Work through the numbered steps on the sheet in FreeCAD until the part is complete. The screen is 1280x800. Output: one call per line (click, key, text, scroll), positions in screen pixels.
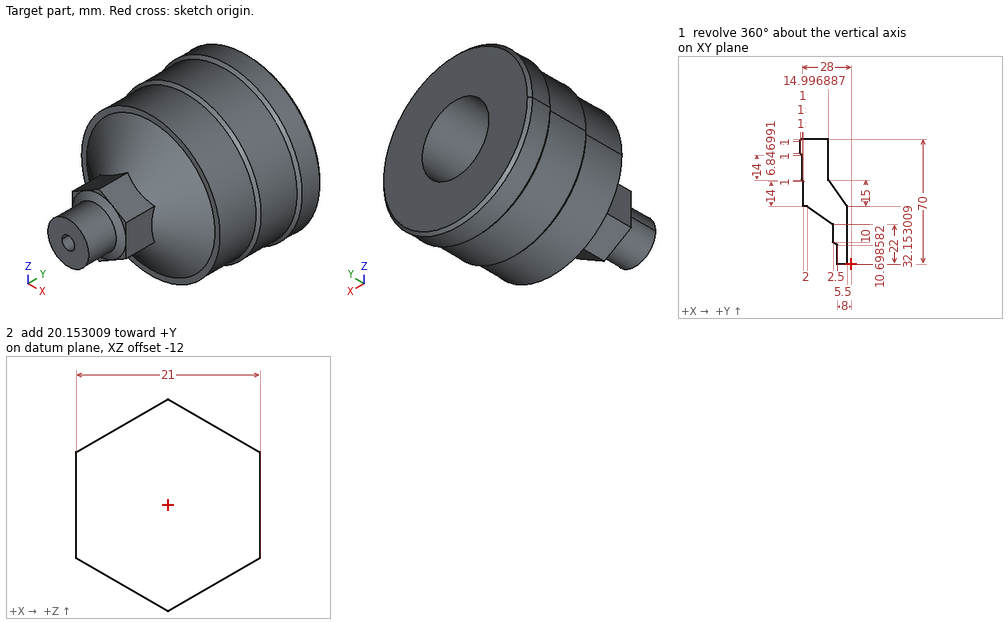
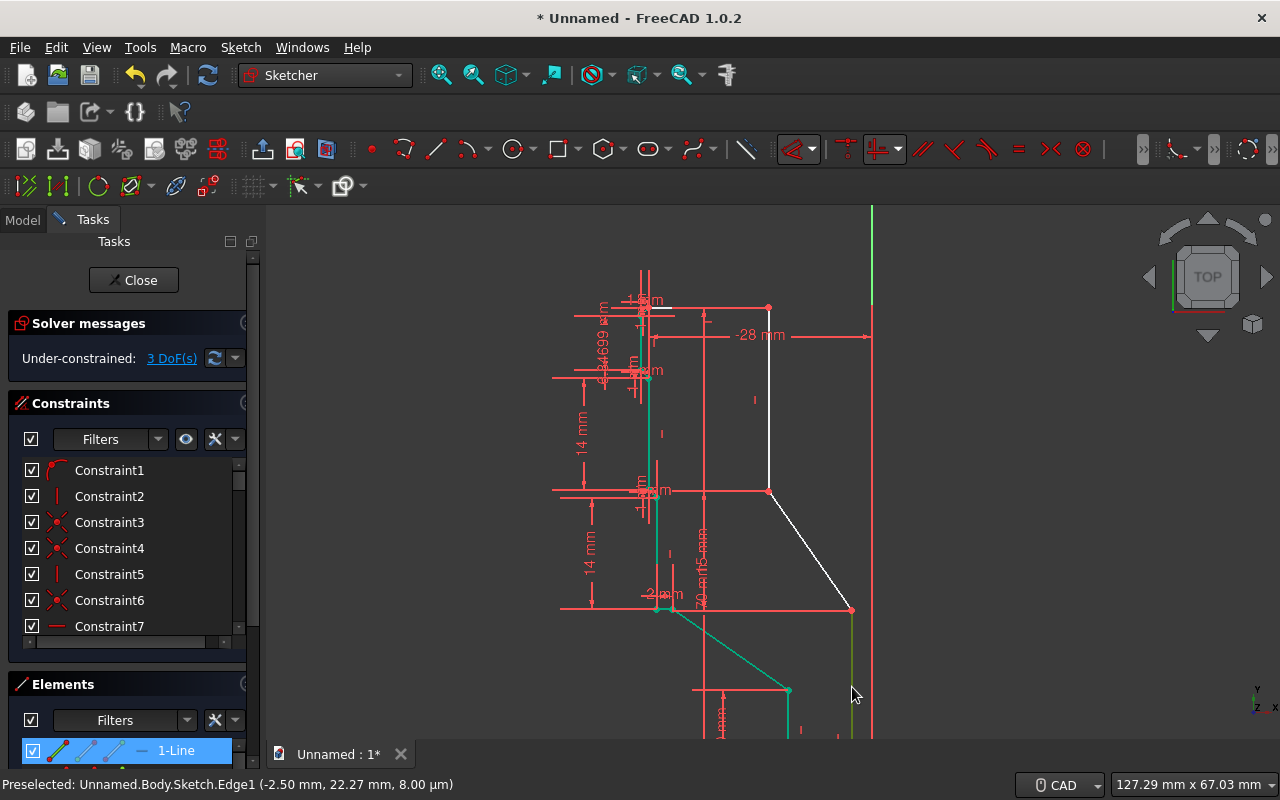
click(814, 150)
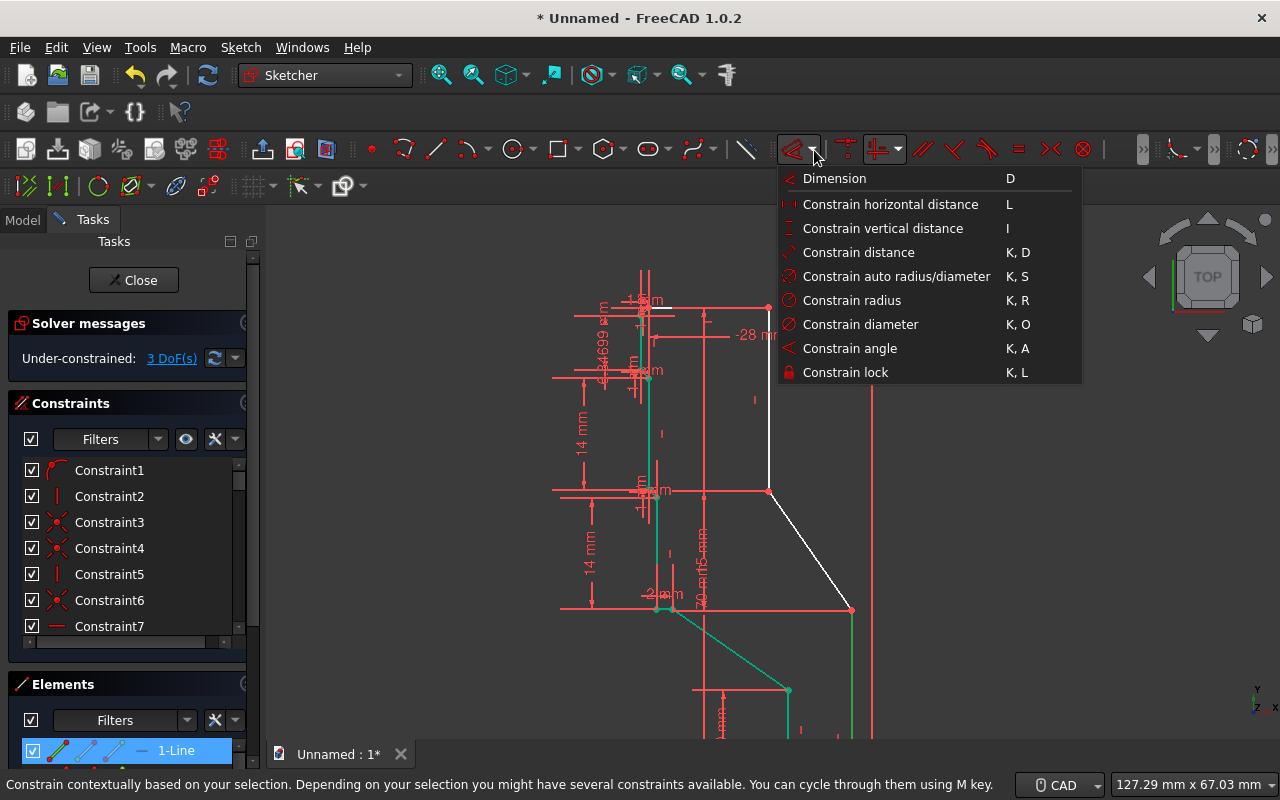
click(930, 228)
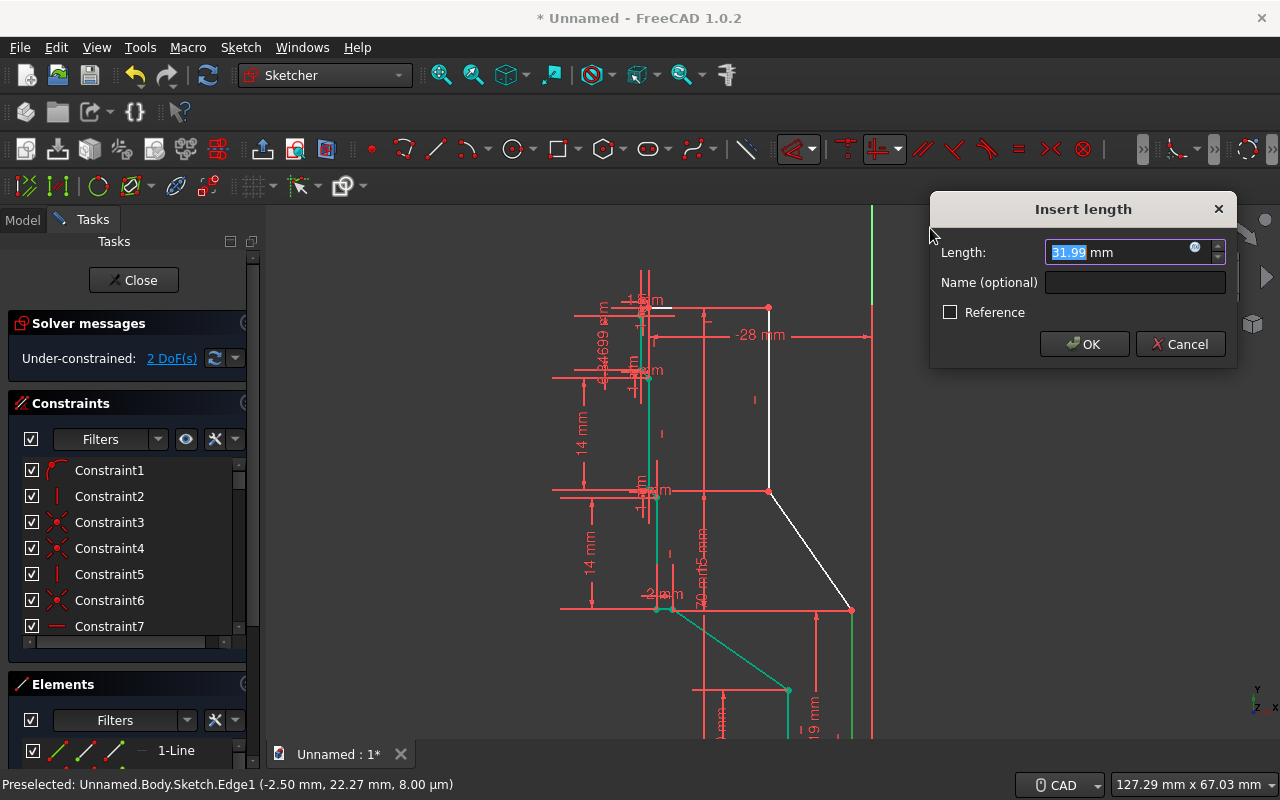
text(32.153009)
key(Return)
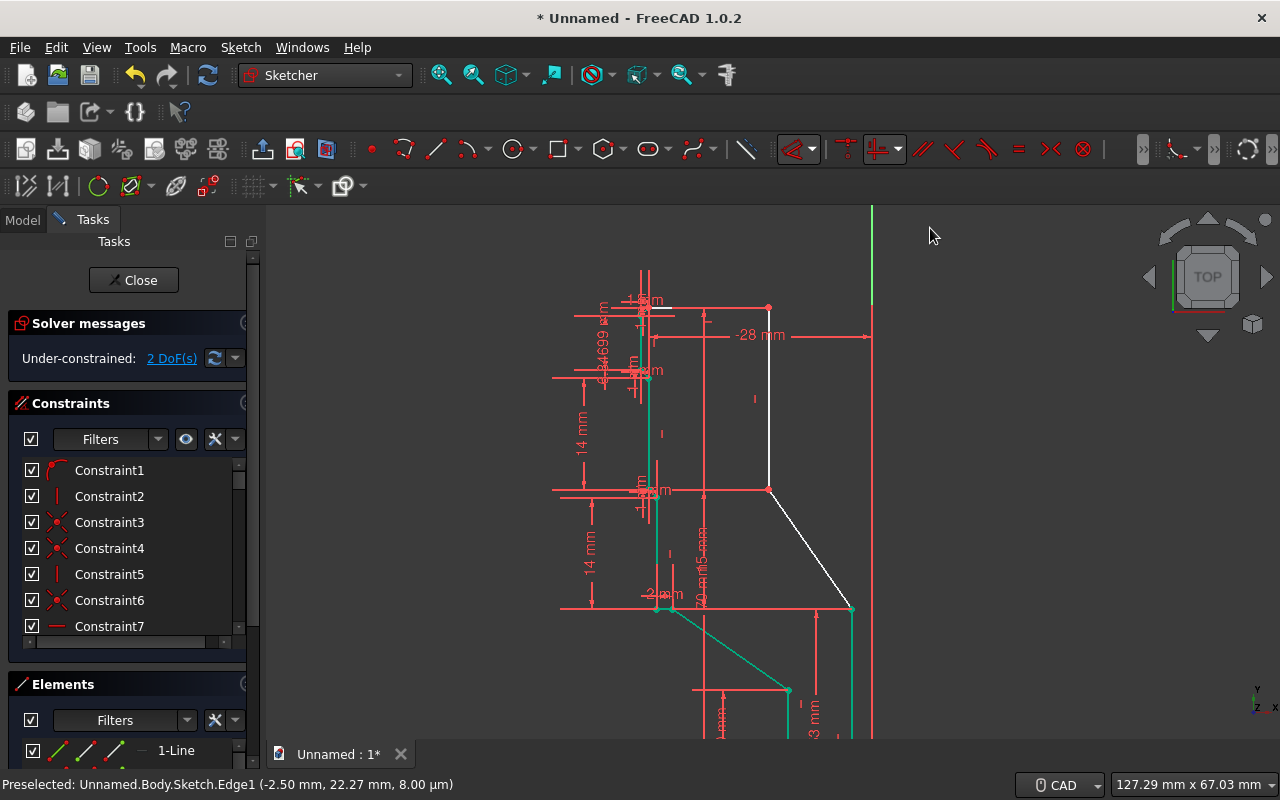
click(733, 308)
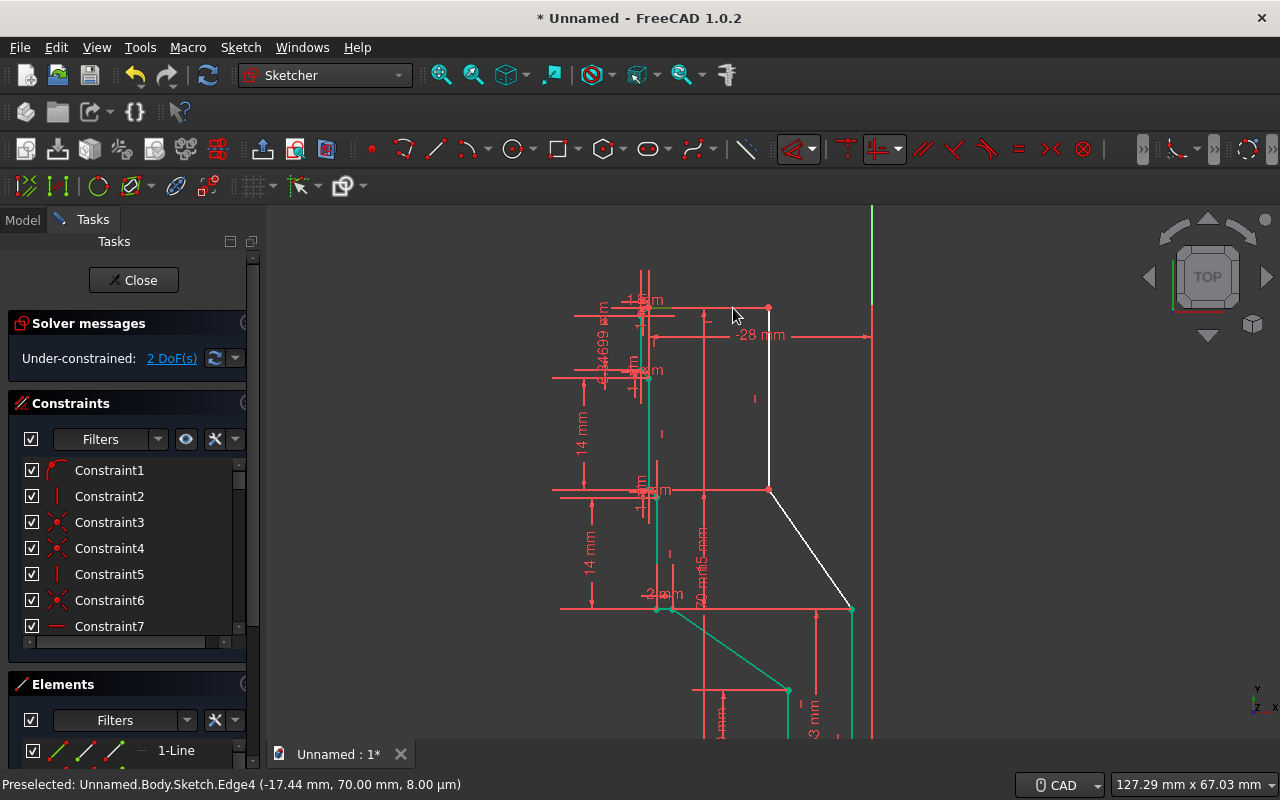
key(l)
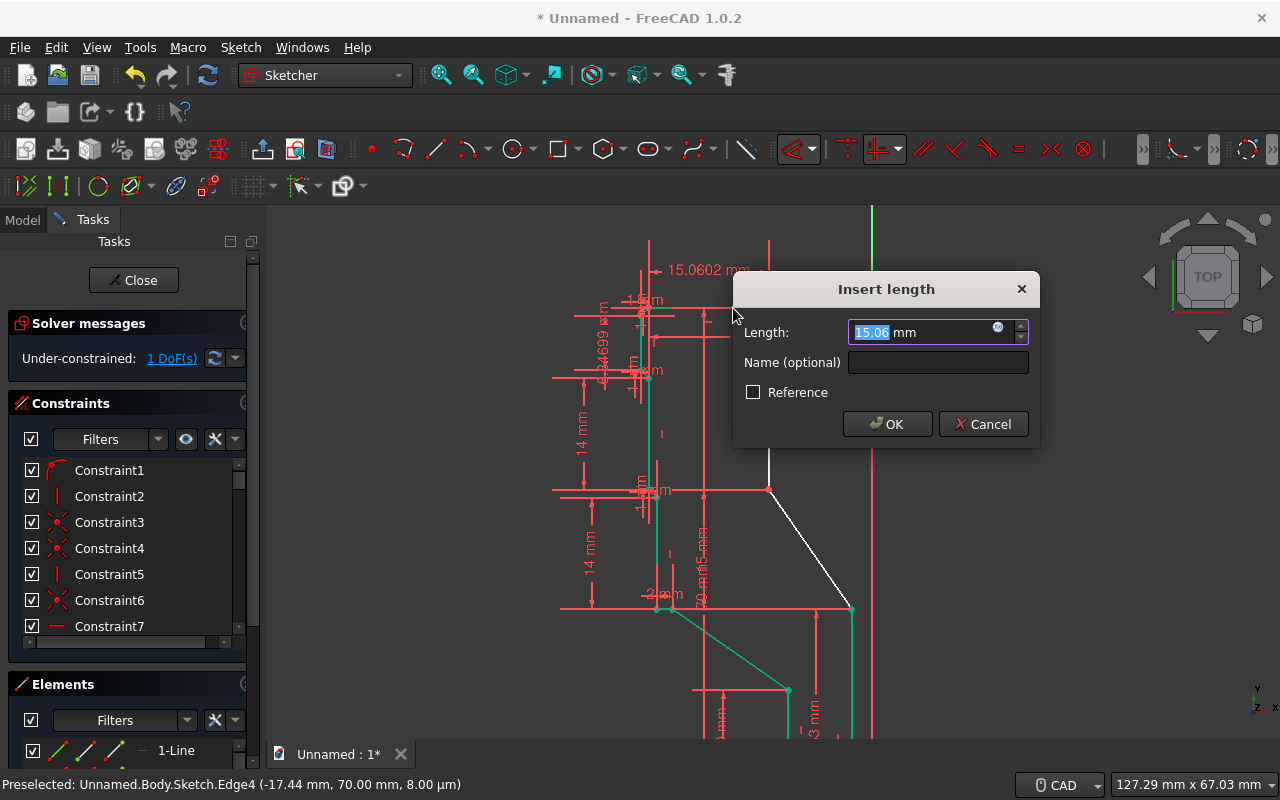
text(14.996887)
key(Return)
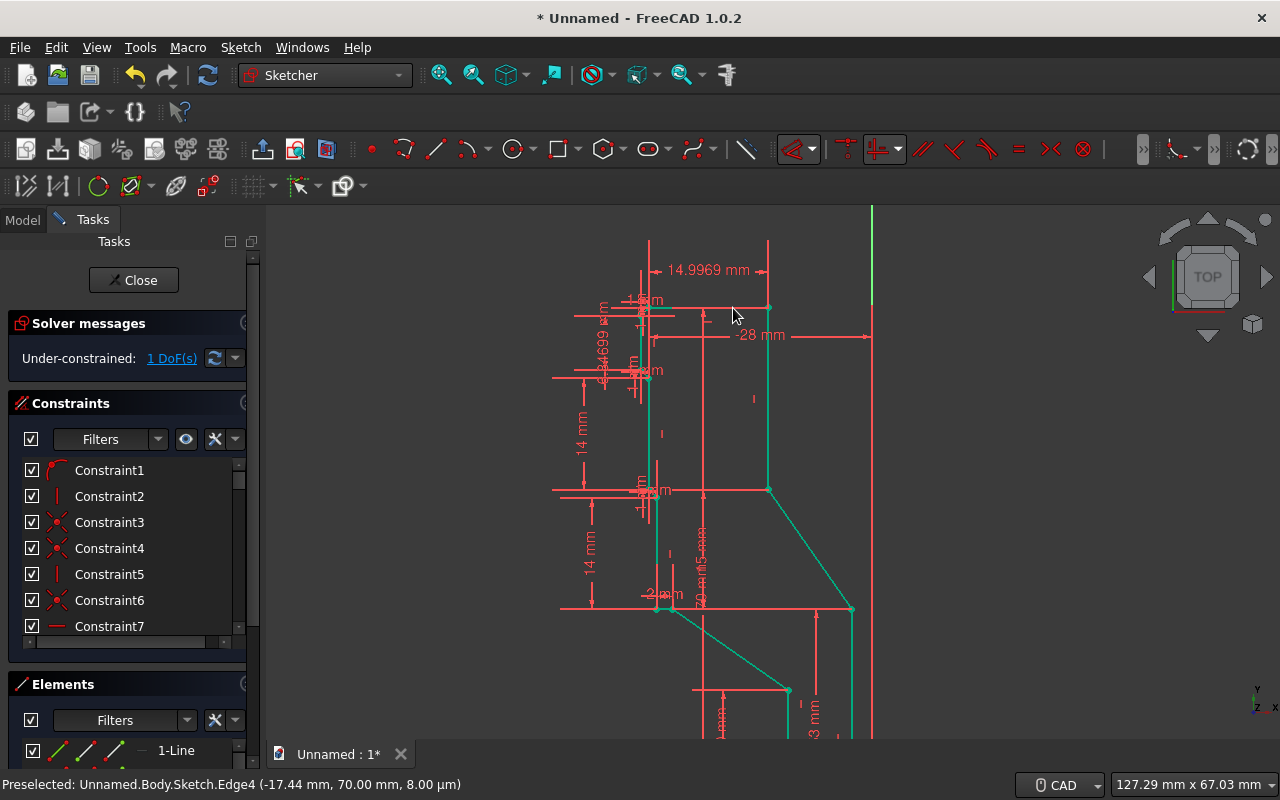
scroll(641, 333, down, 3)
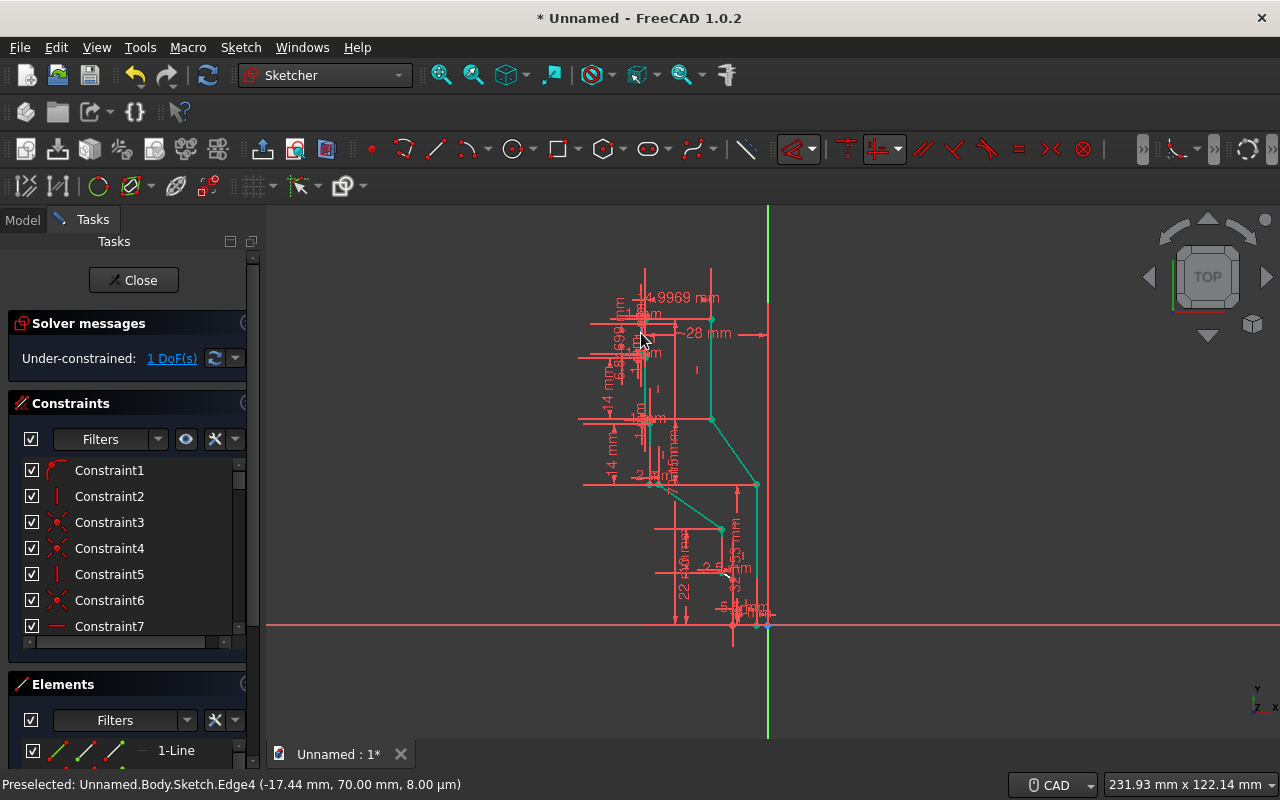
click(733, 593)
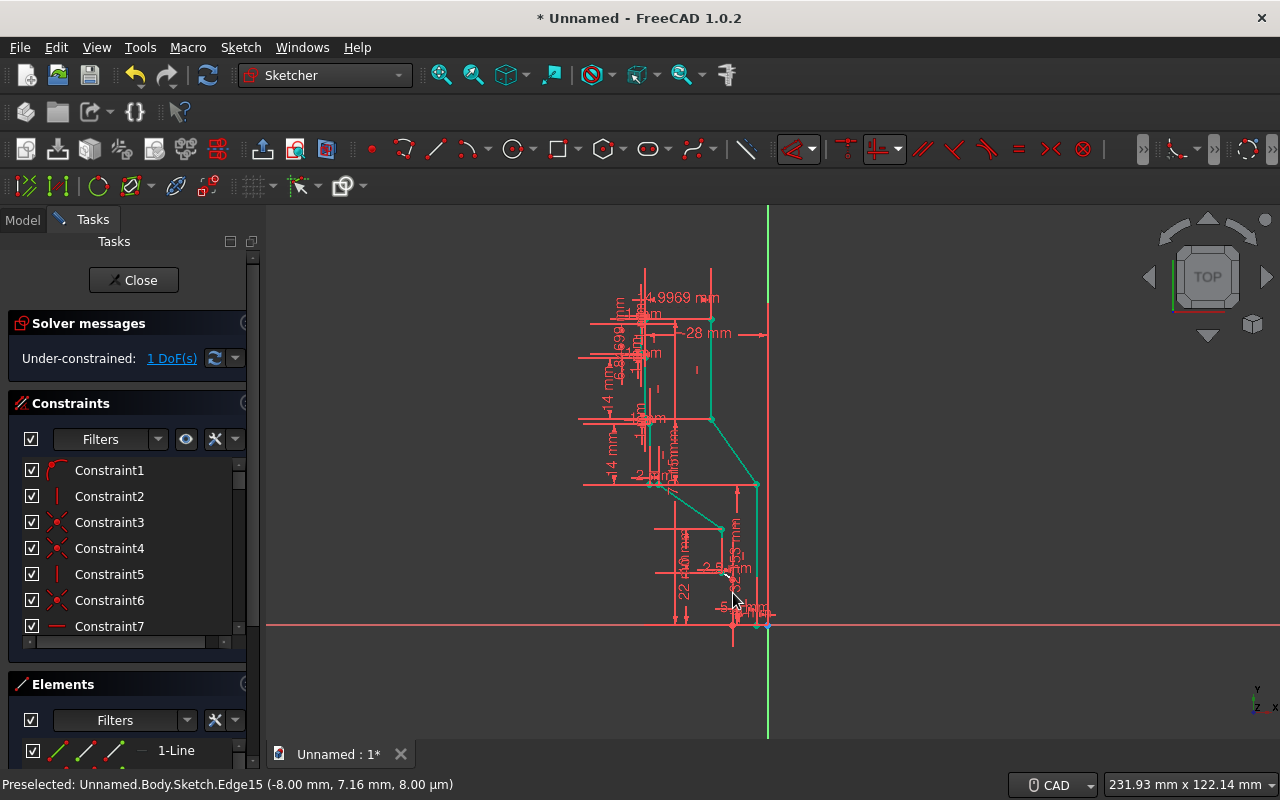
click(814, 150)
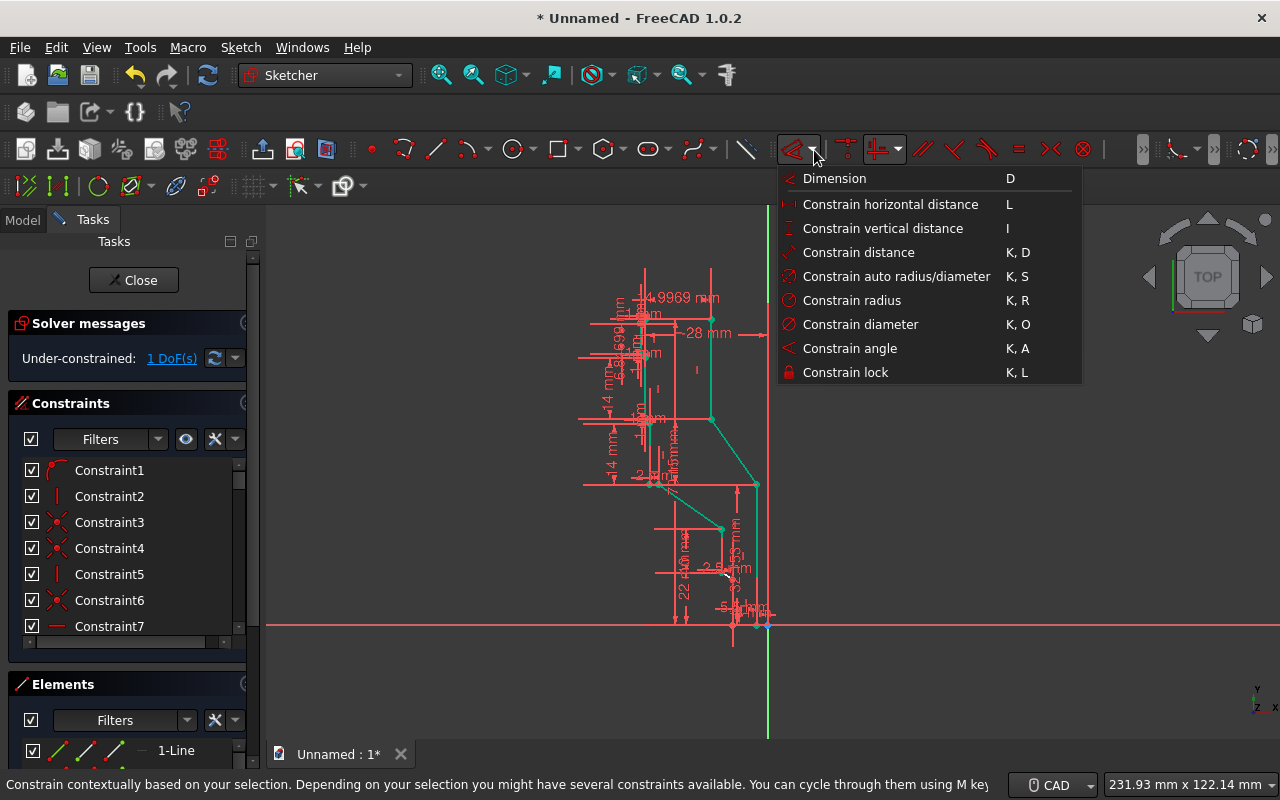
click(930, 228)